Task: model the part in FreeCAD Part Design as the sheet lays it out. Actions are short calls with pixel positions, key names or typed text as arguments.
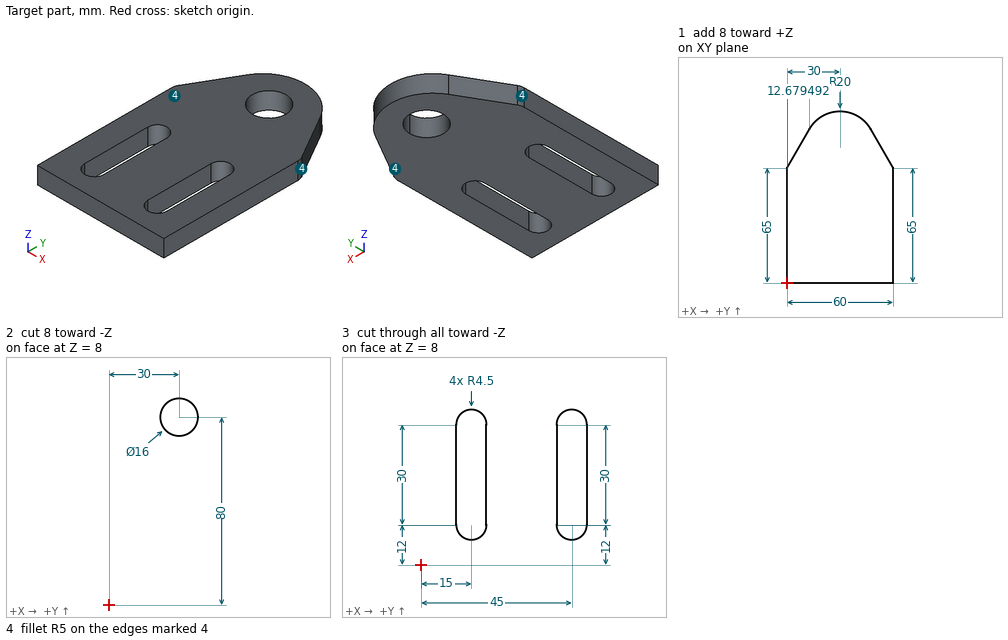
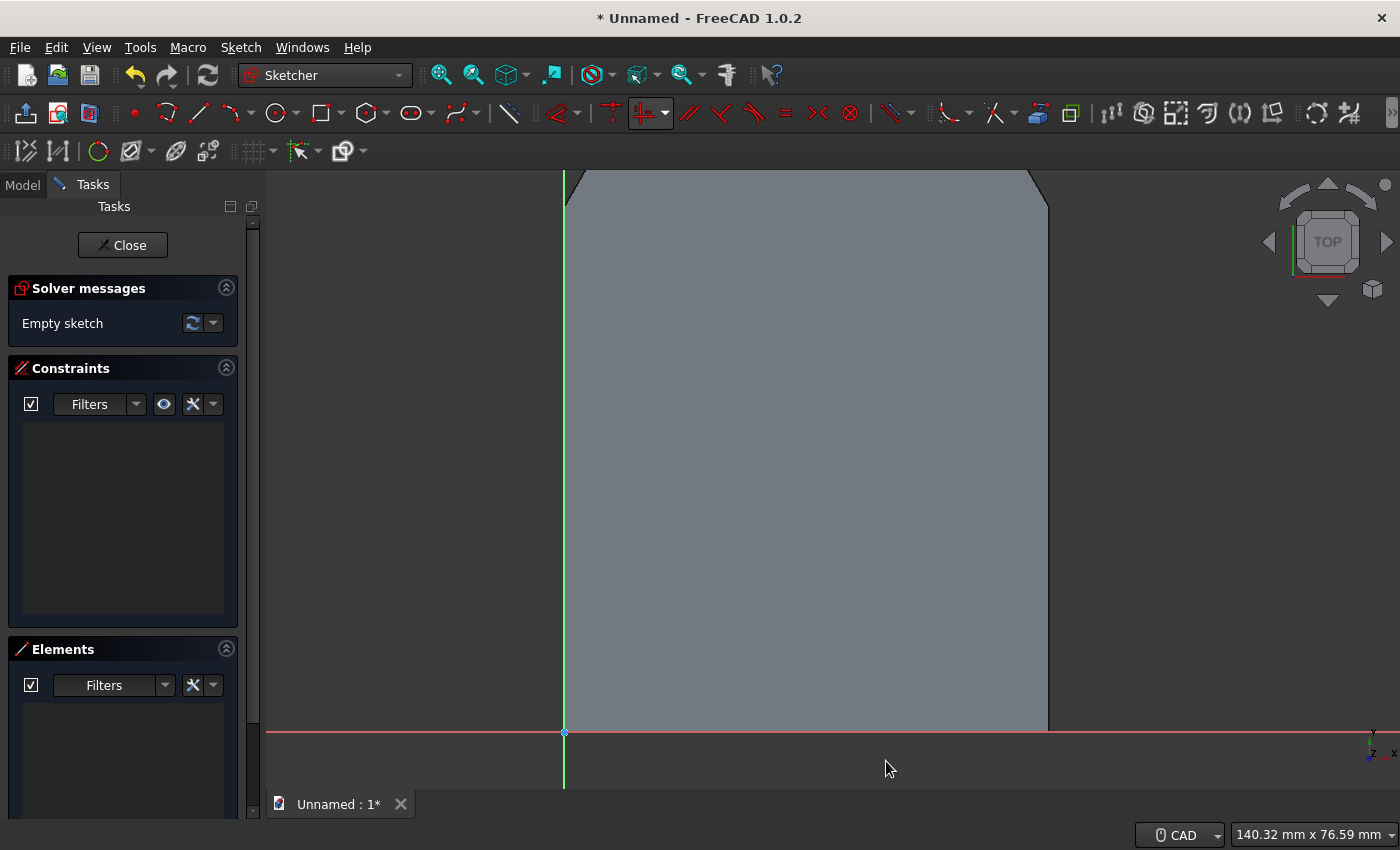
click(685, 635)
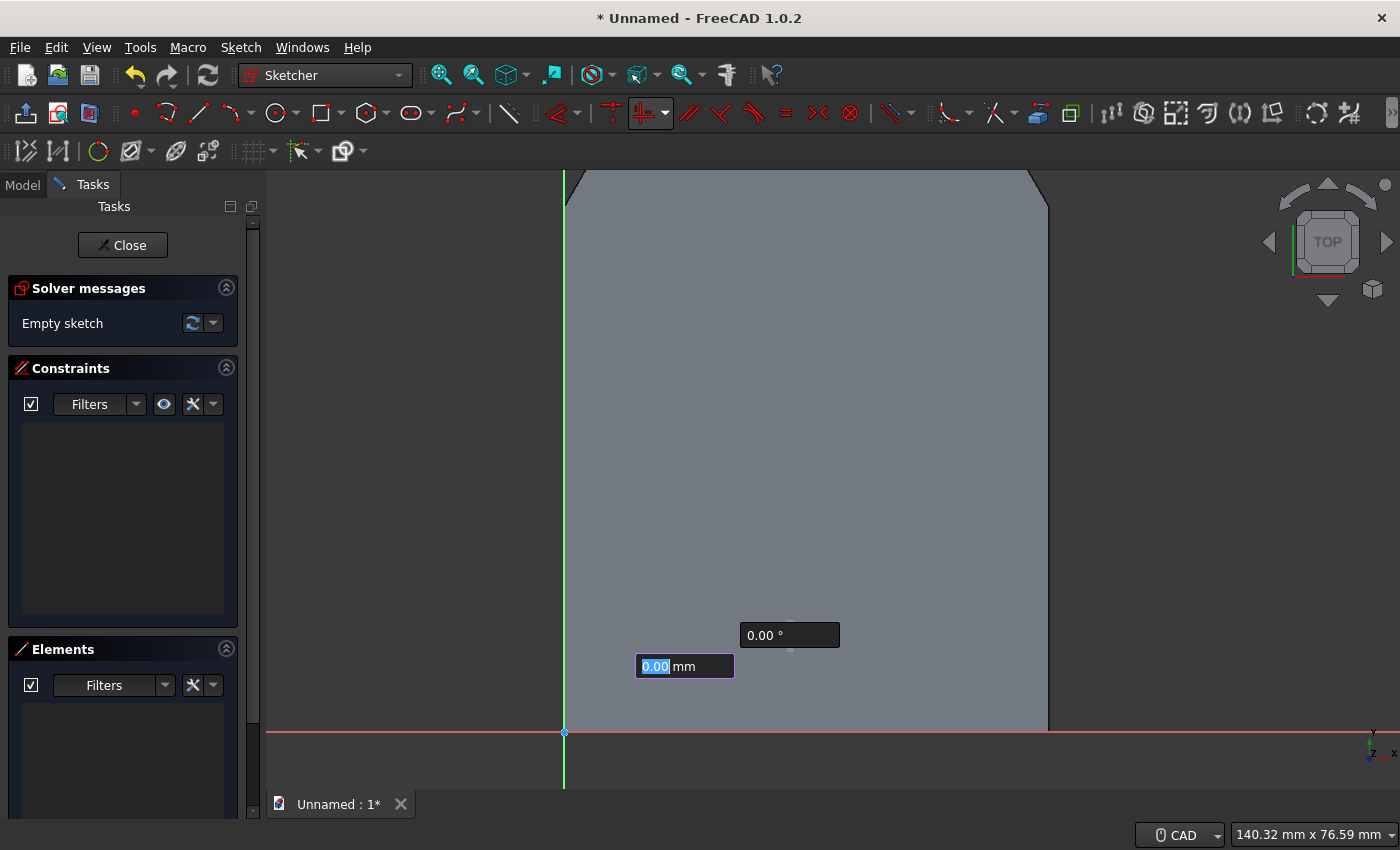
click(685, 393)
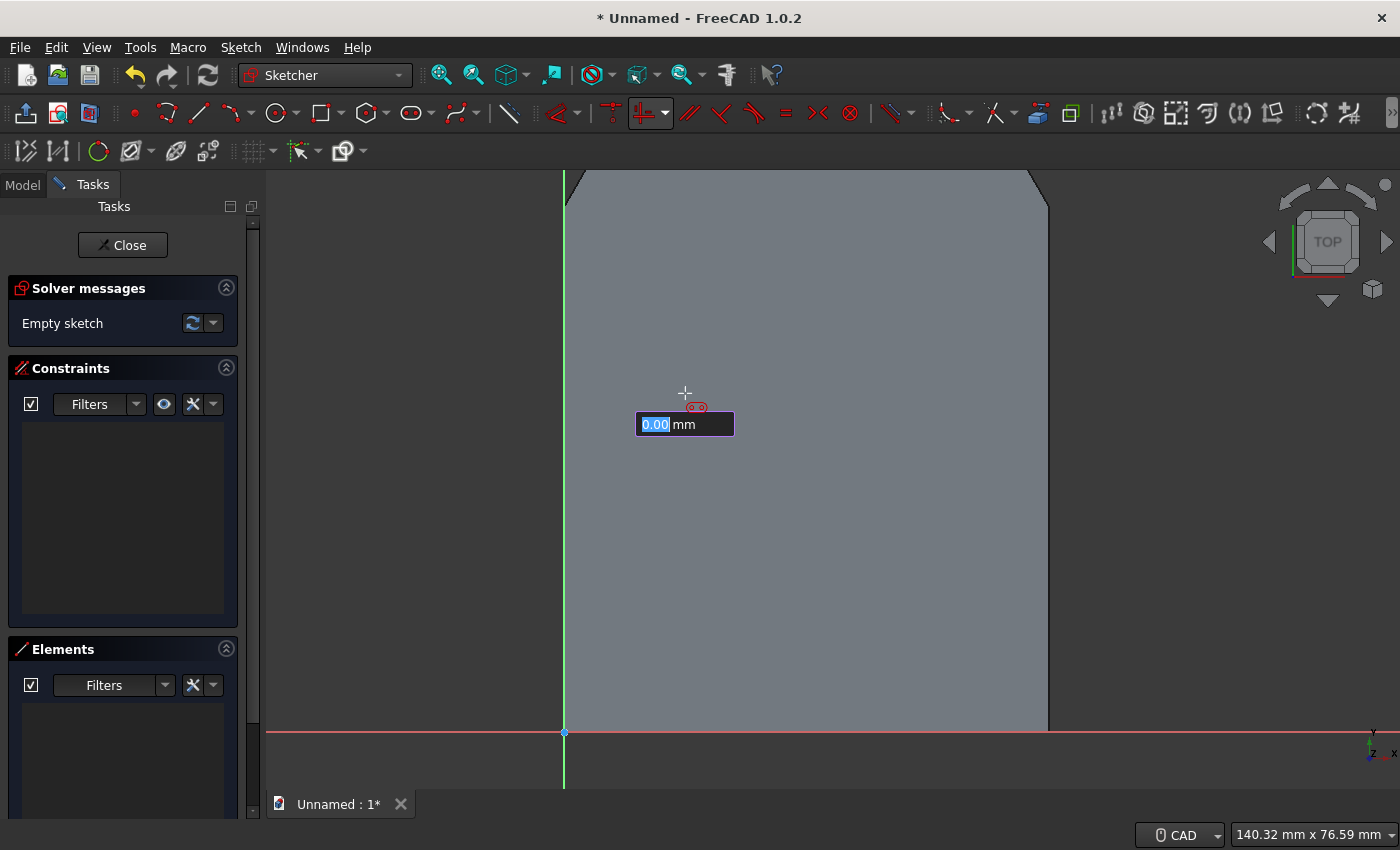
click(649, 514)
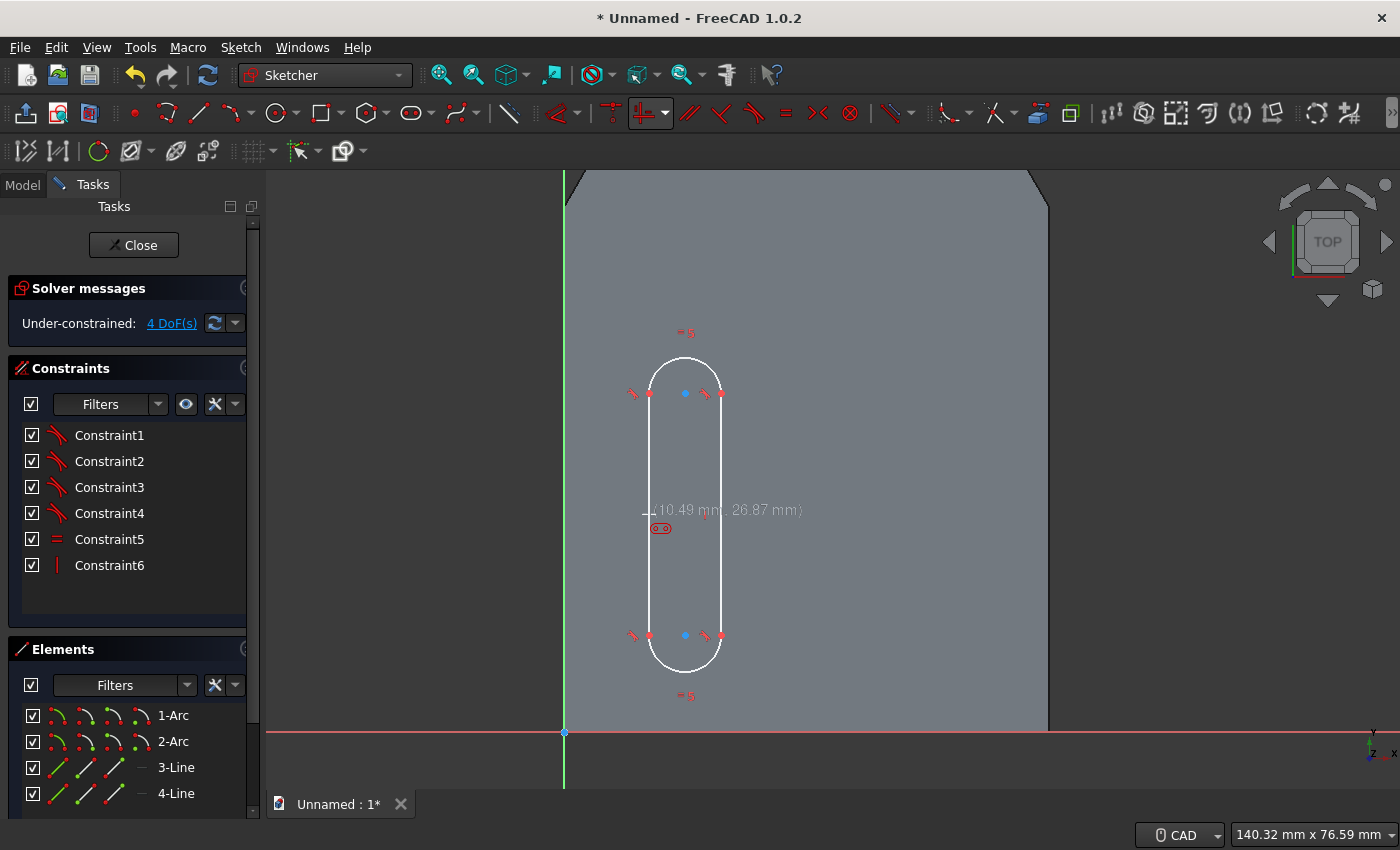
click(928, 635)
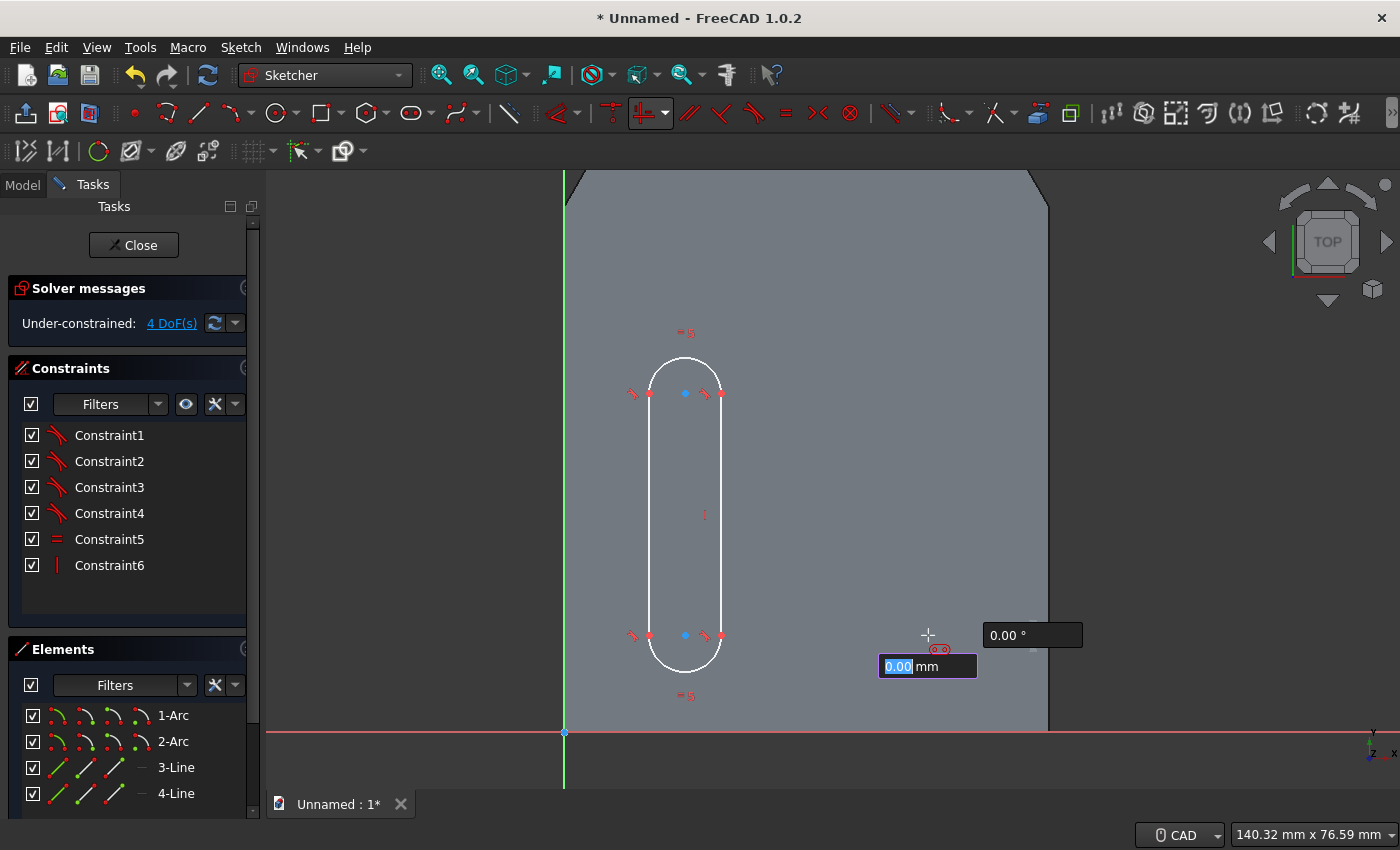
click(928, 393)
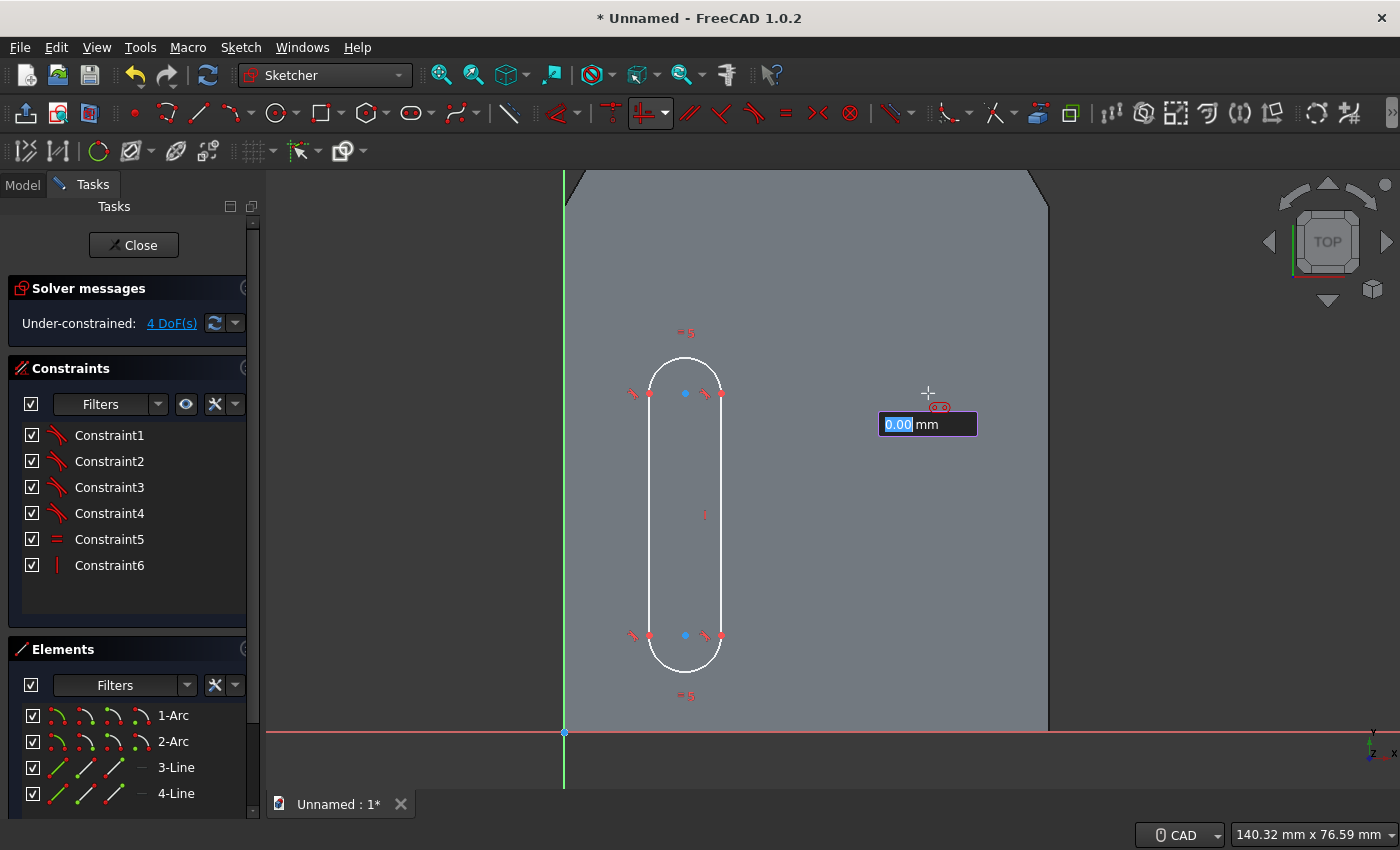
click(964, 514)
key(Escape)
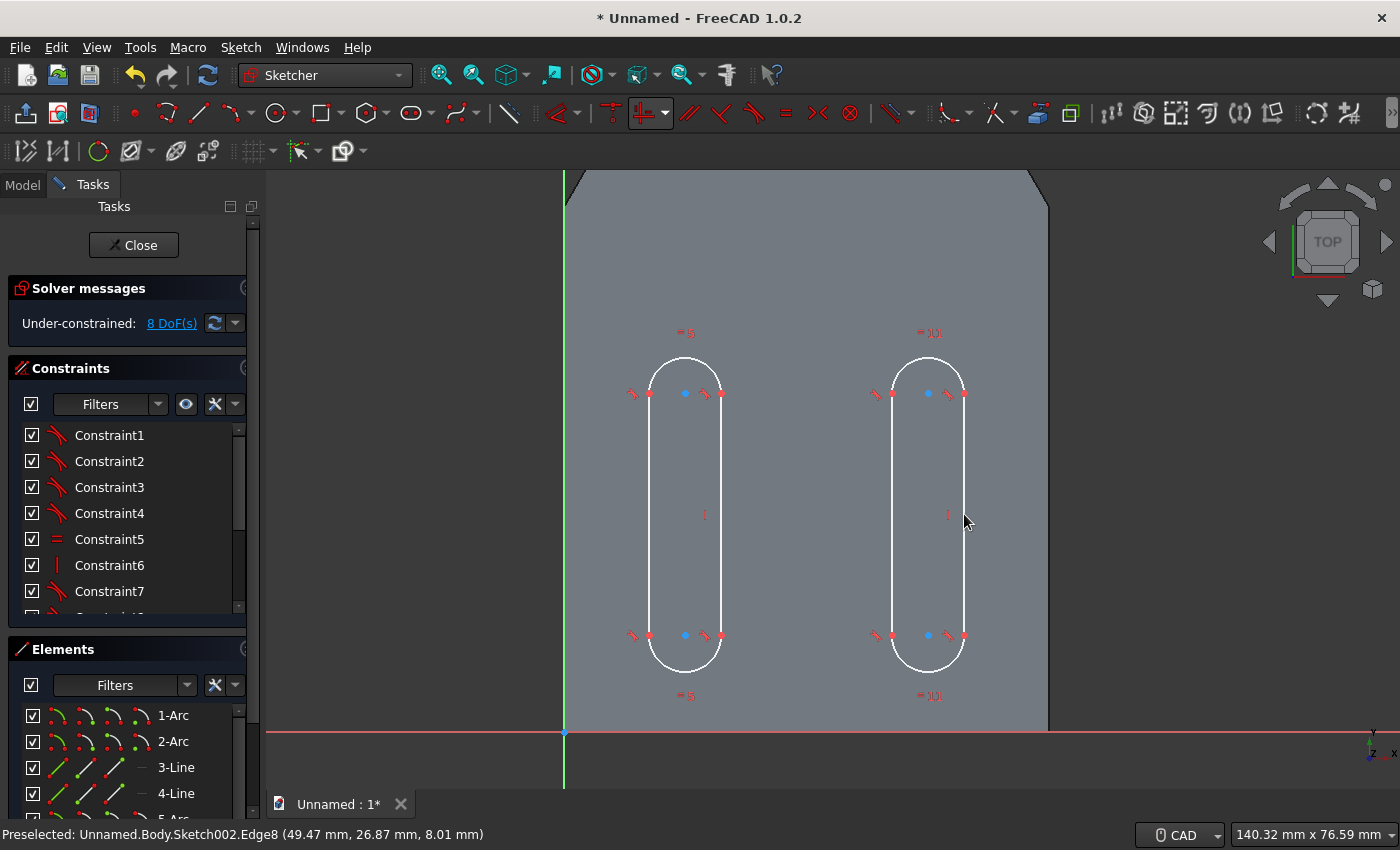
click(664, 665)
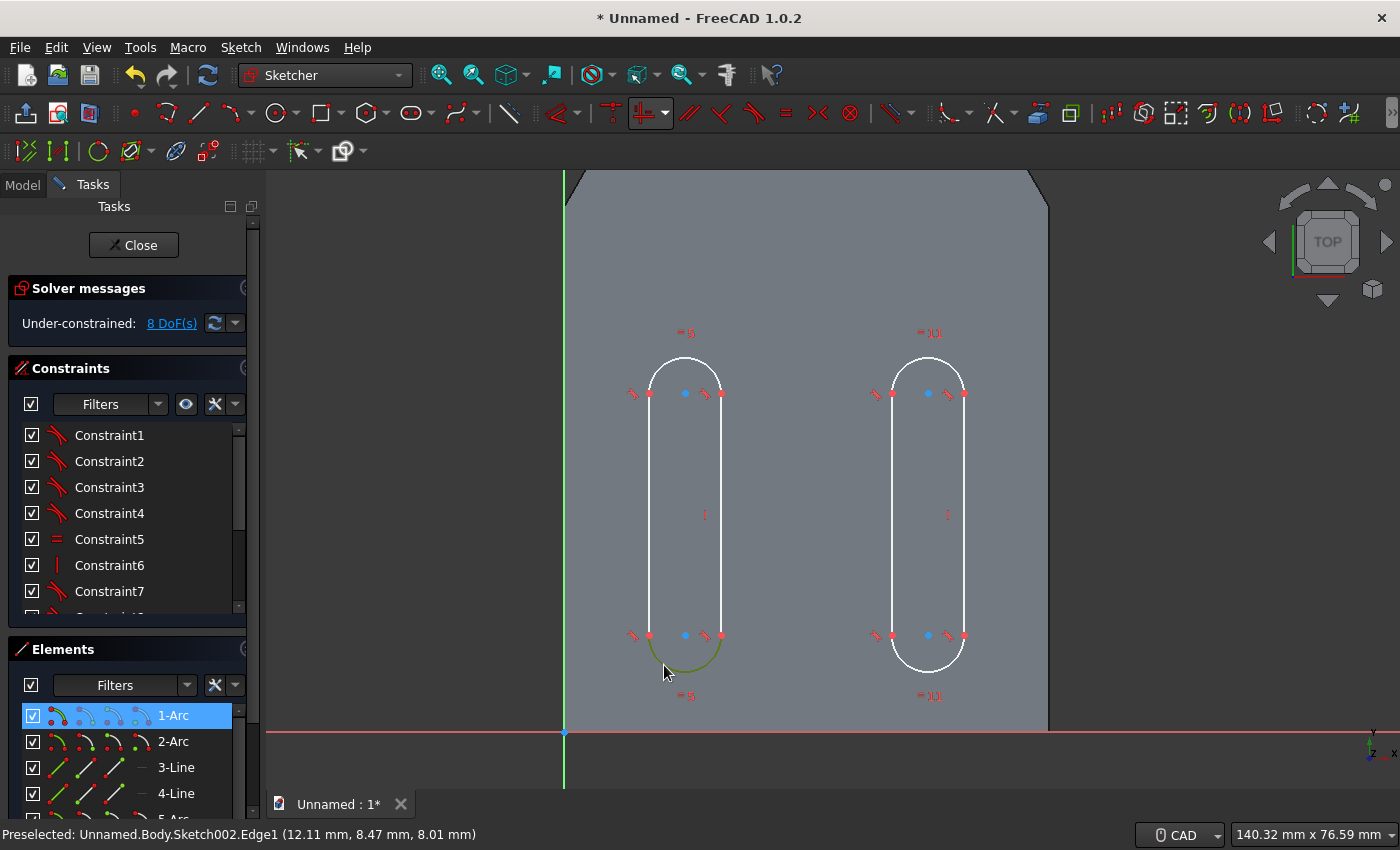
click(907, 665)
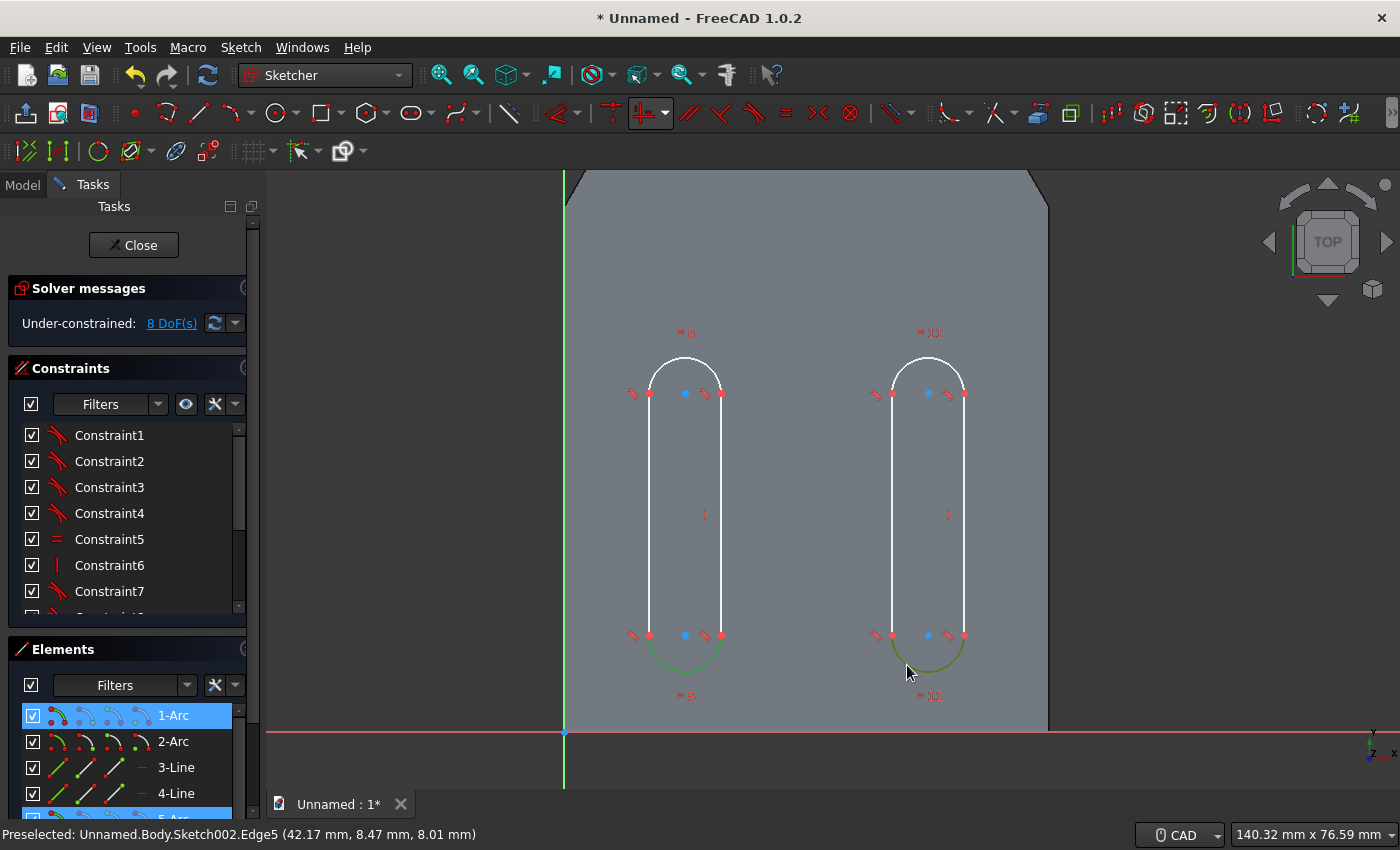
key(e)